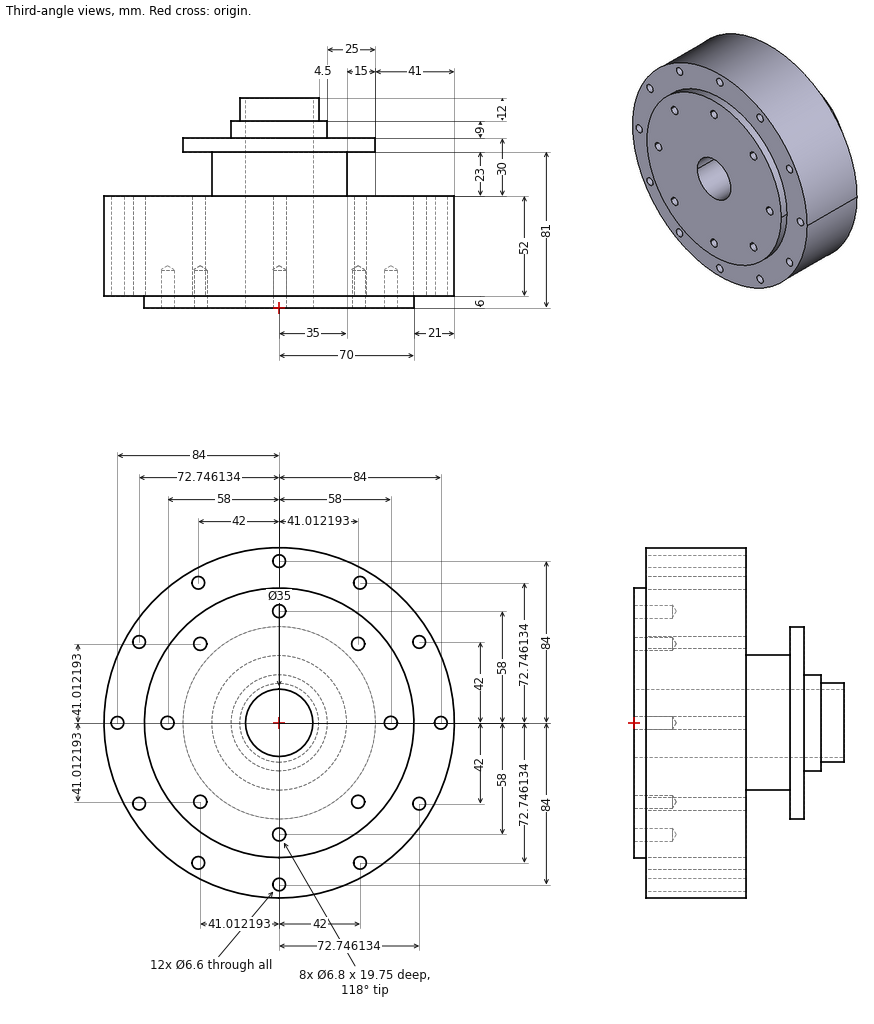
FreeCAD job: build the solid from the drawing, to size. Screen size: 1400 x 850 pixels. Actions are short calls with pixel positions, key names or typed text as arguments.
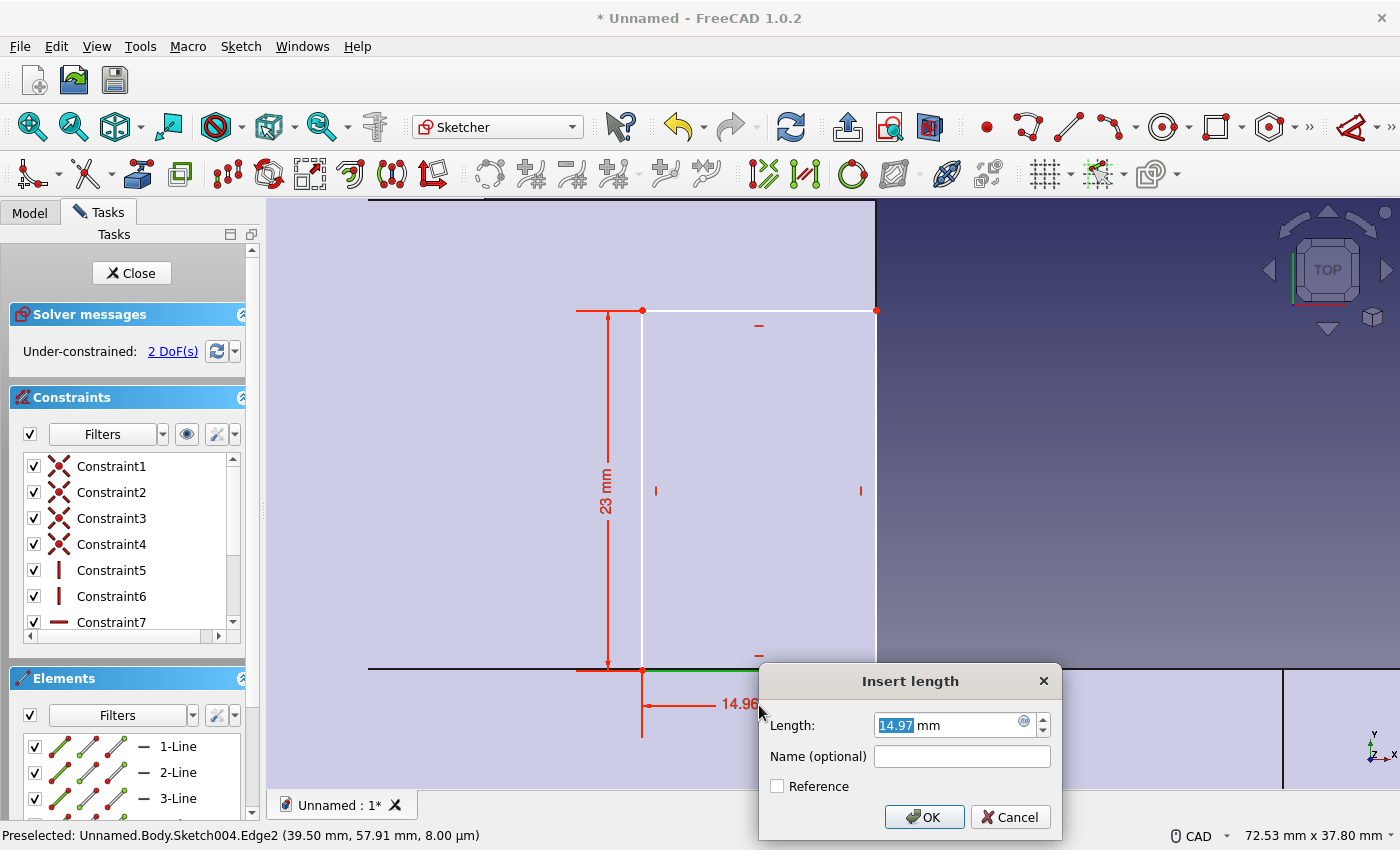
text(15)
key(Return)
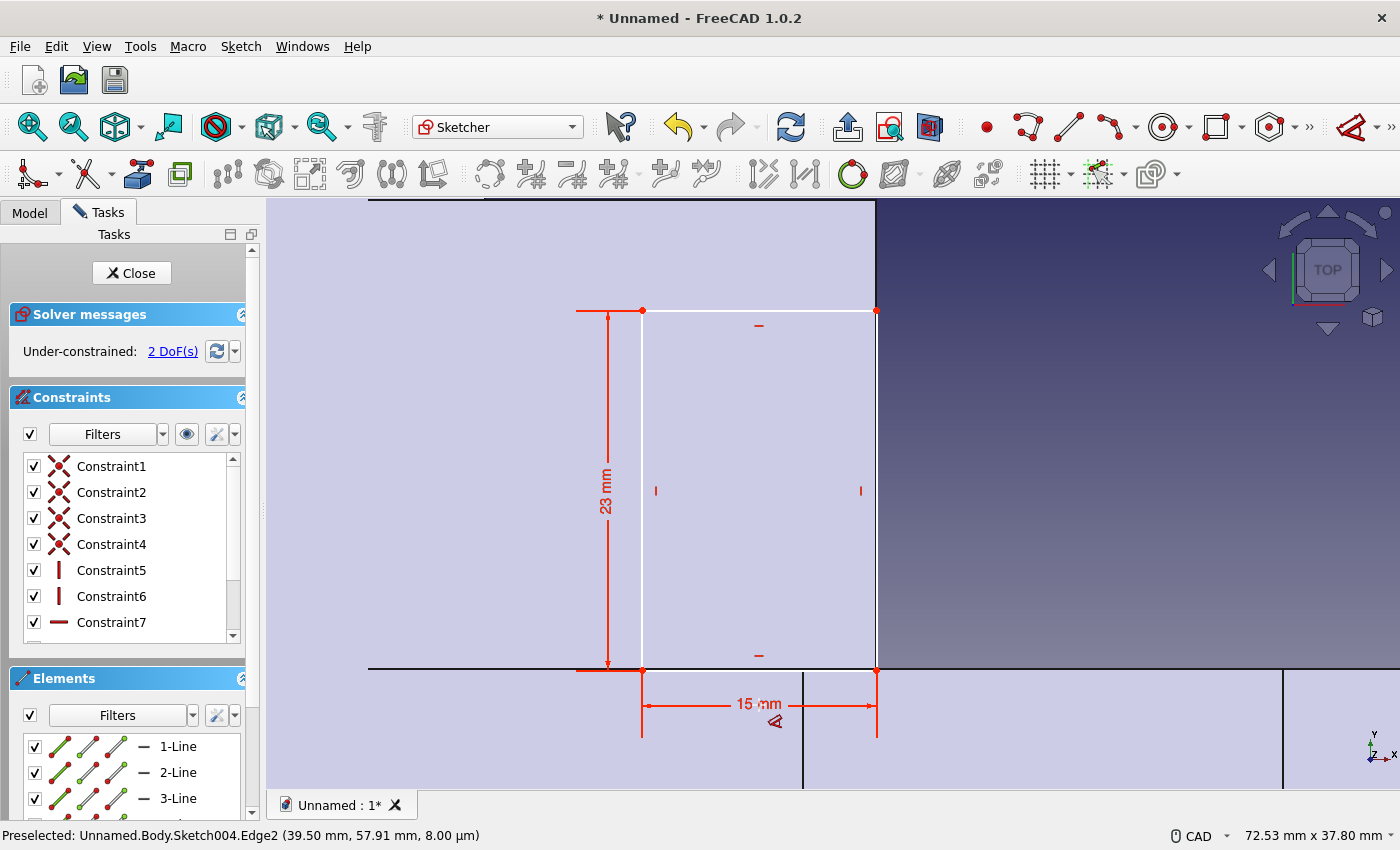
click(642, 311)
click(468, 277)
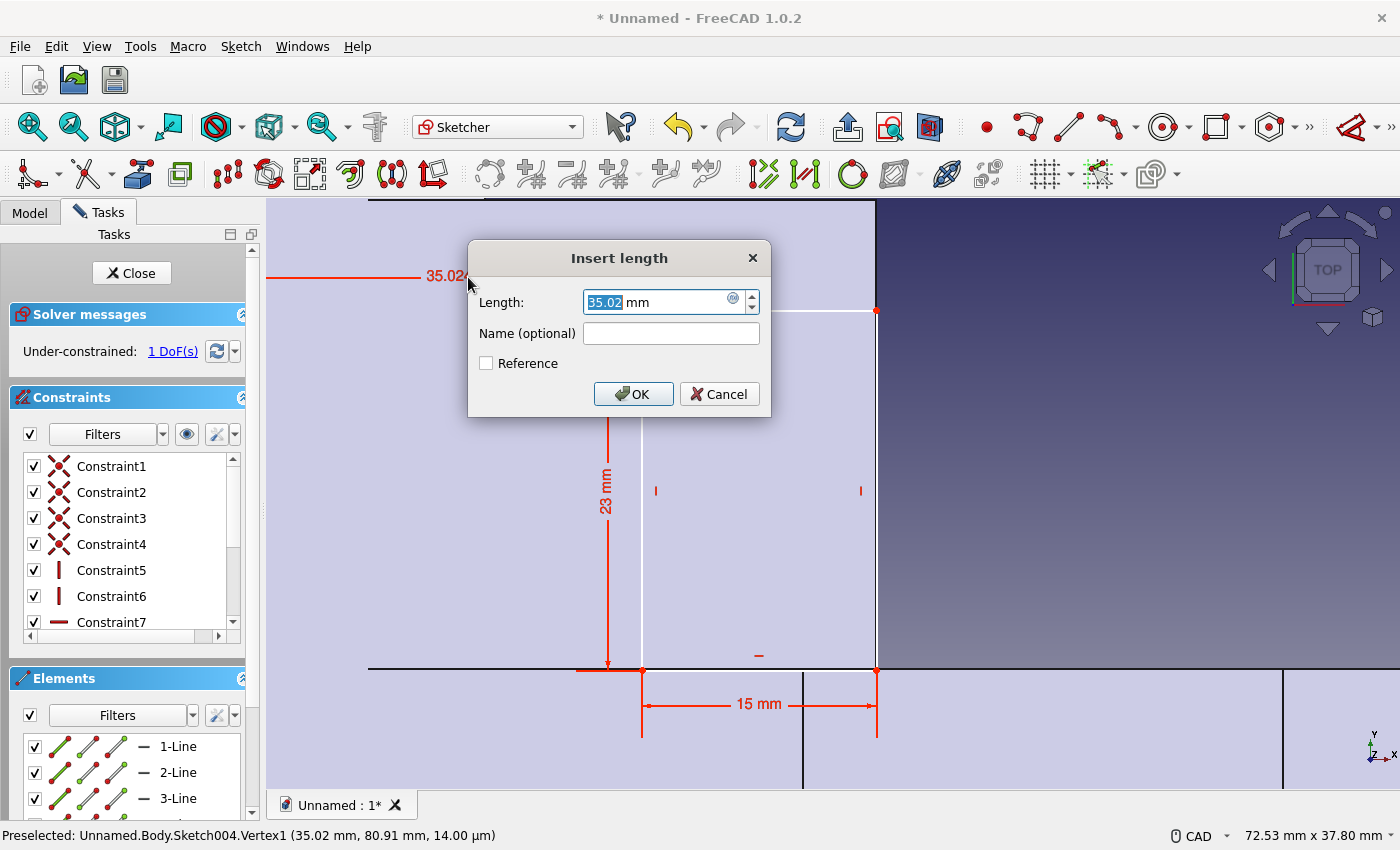
text(35)
key(Return)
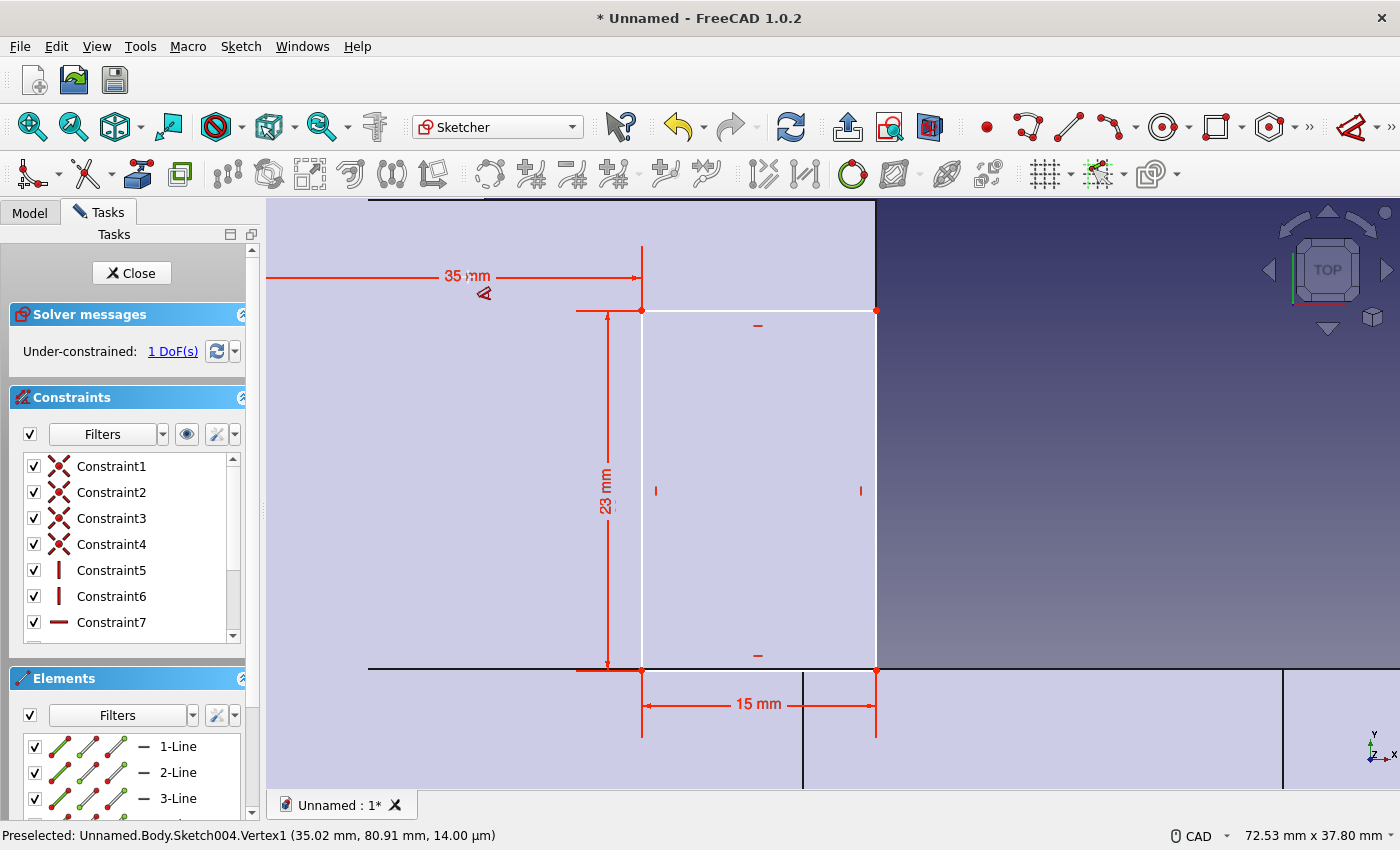
click(642, 311)
click(676, 536)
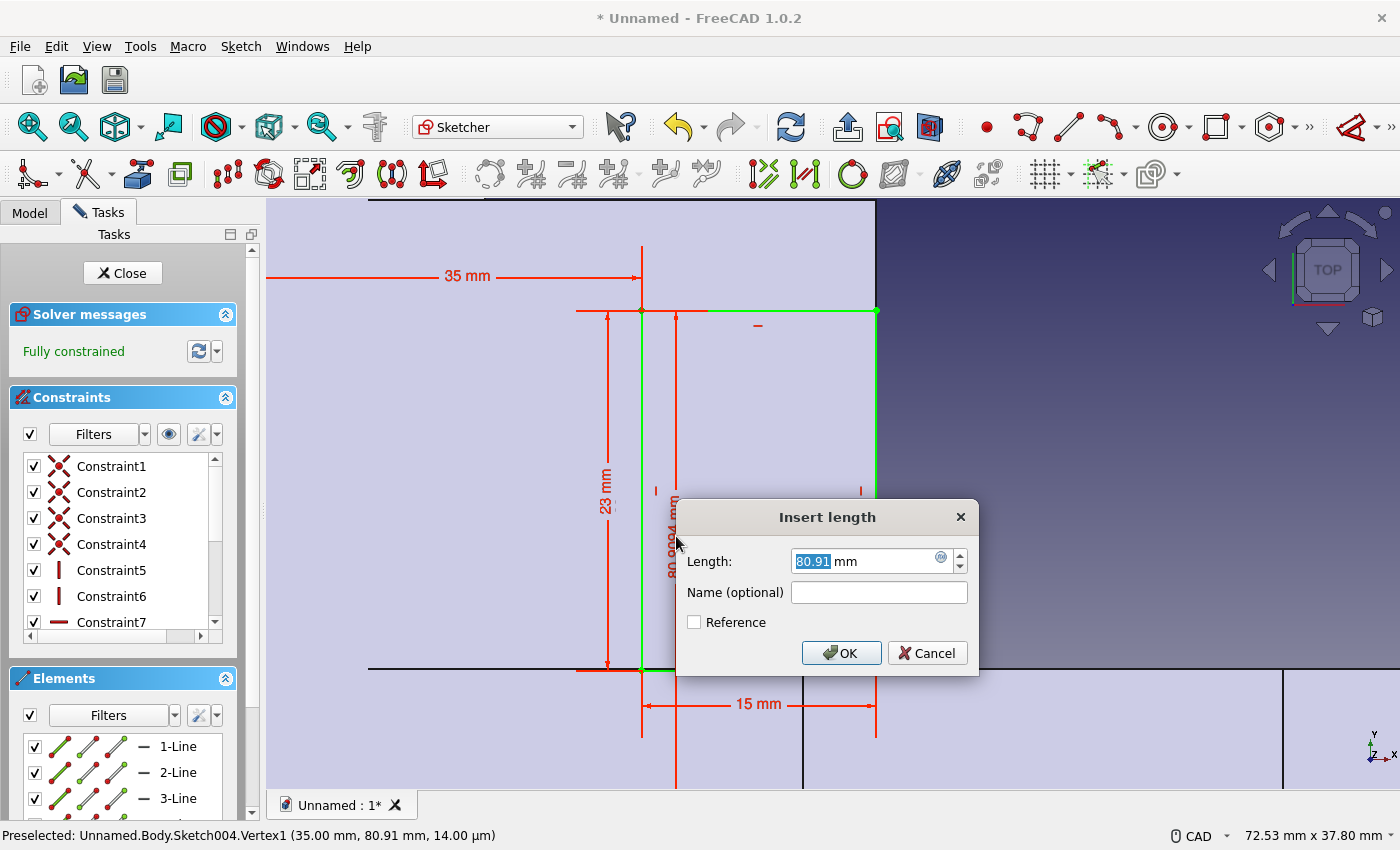
text(81)
key(Return)
key(Escape)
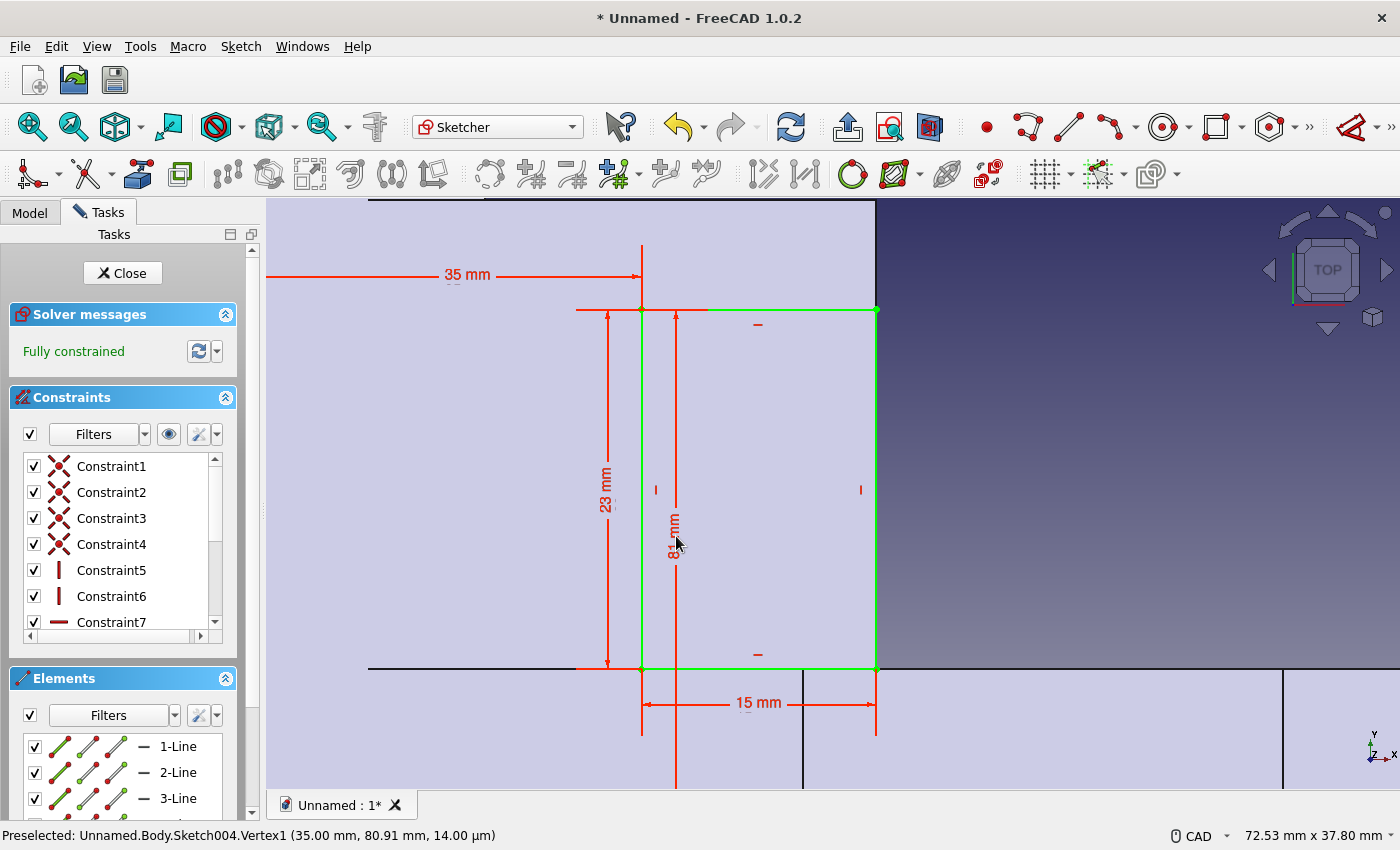
click(123, 273)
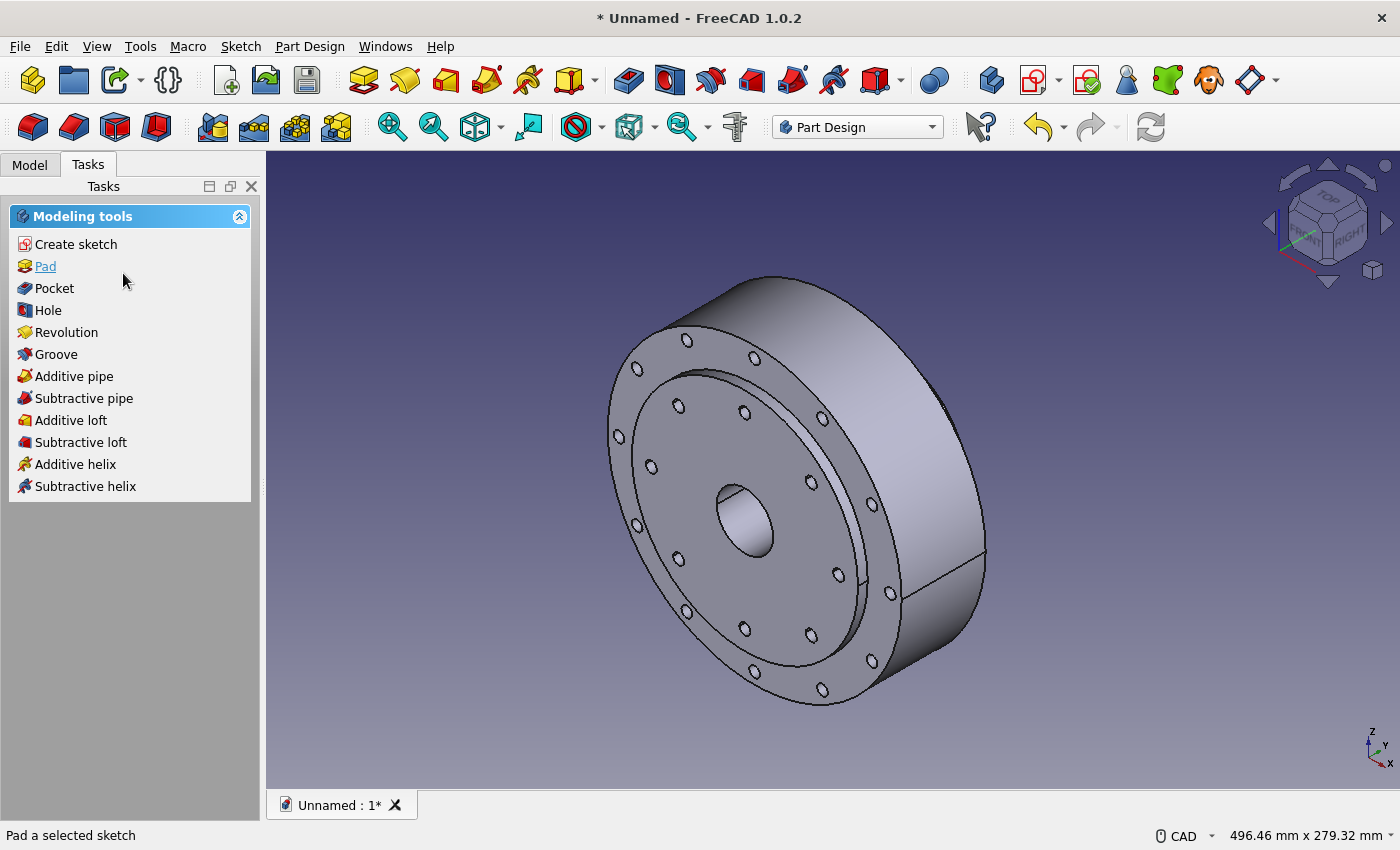
click(711, 80)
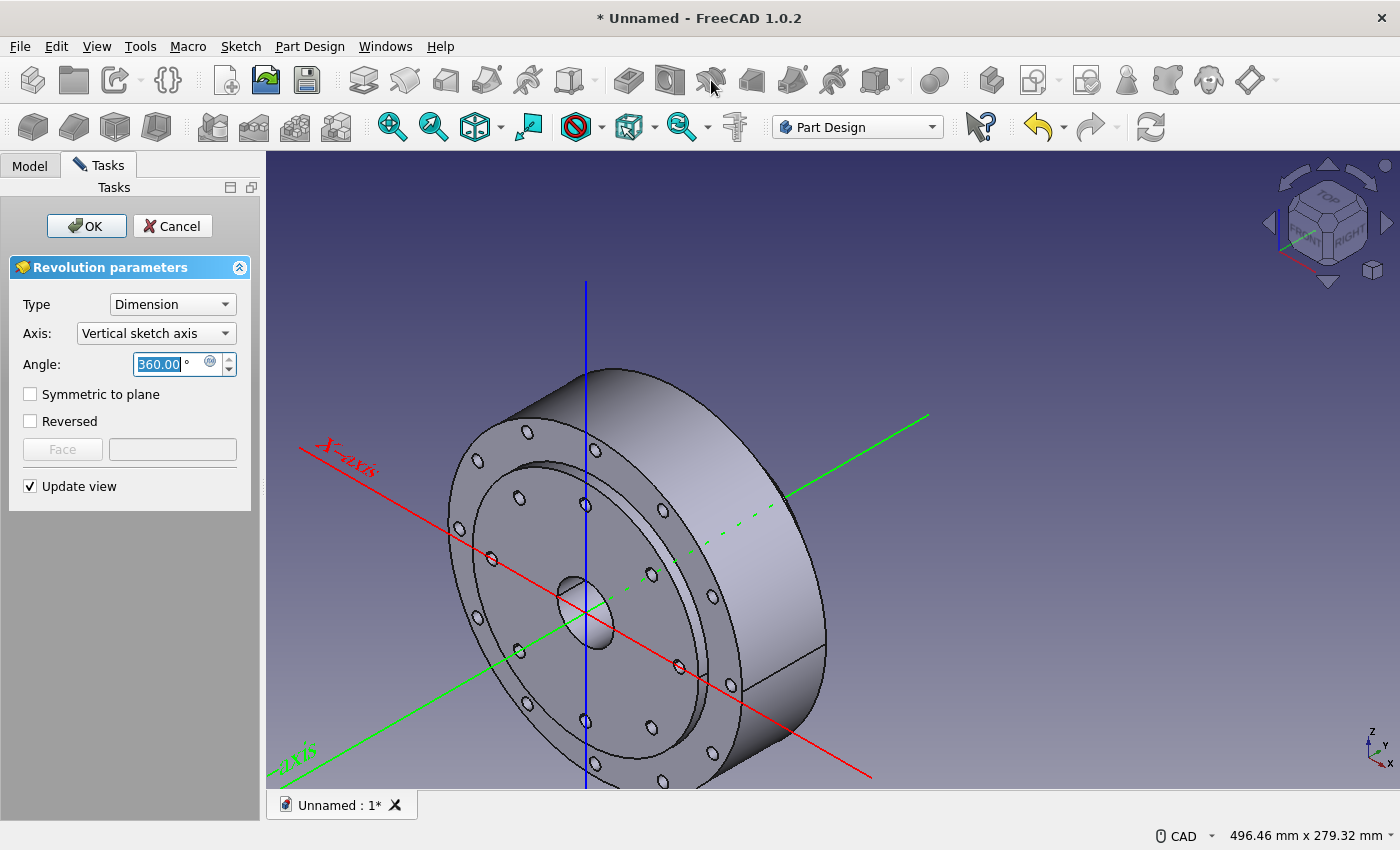
click(87, 226)